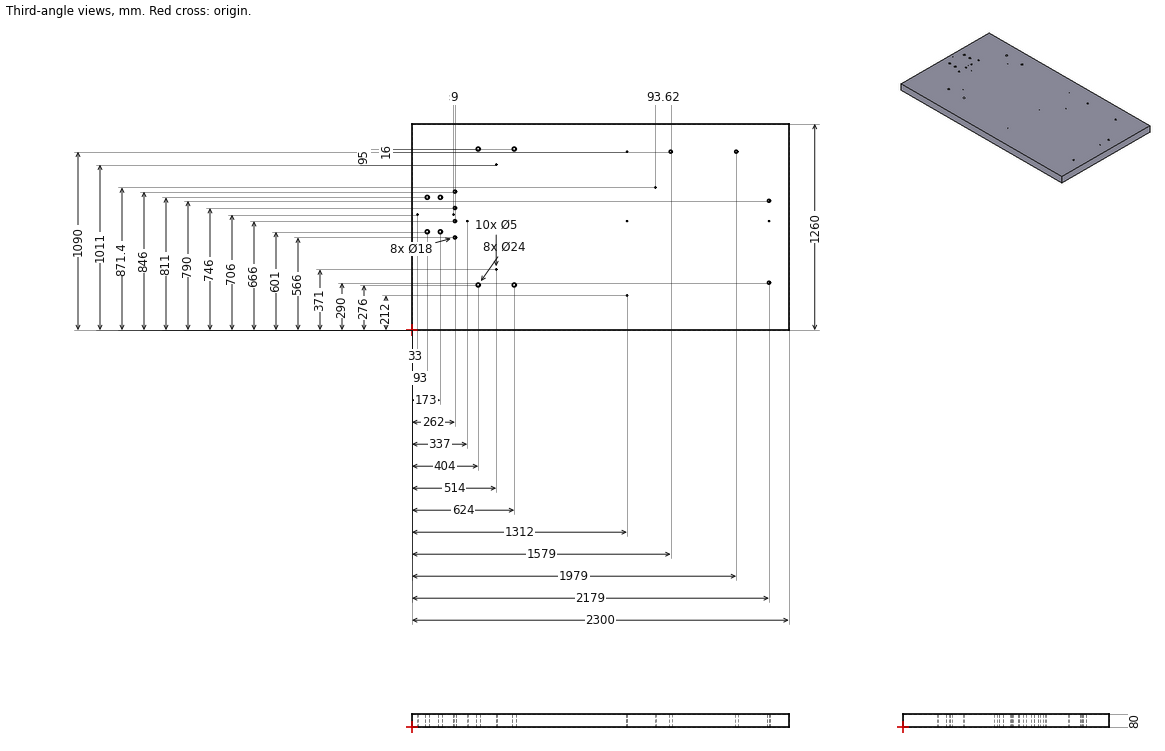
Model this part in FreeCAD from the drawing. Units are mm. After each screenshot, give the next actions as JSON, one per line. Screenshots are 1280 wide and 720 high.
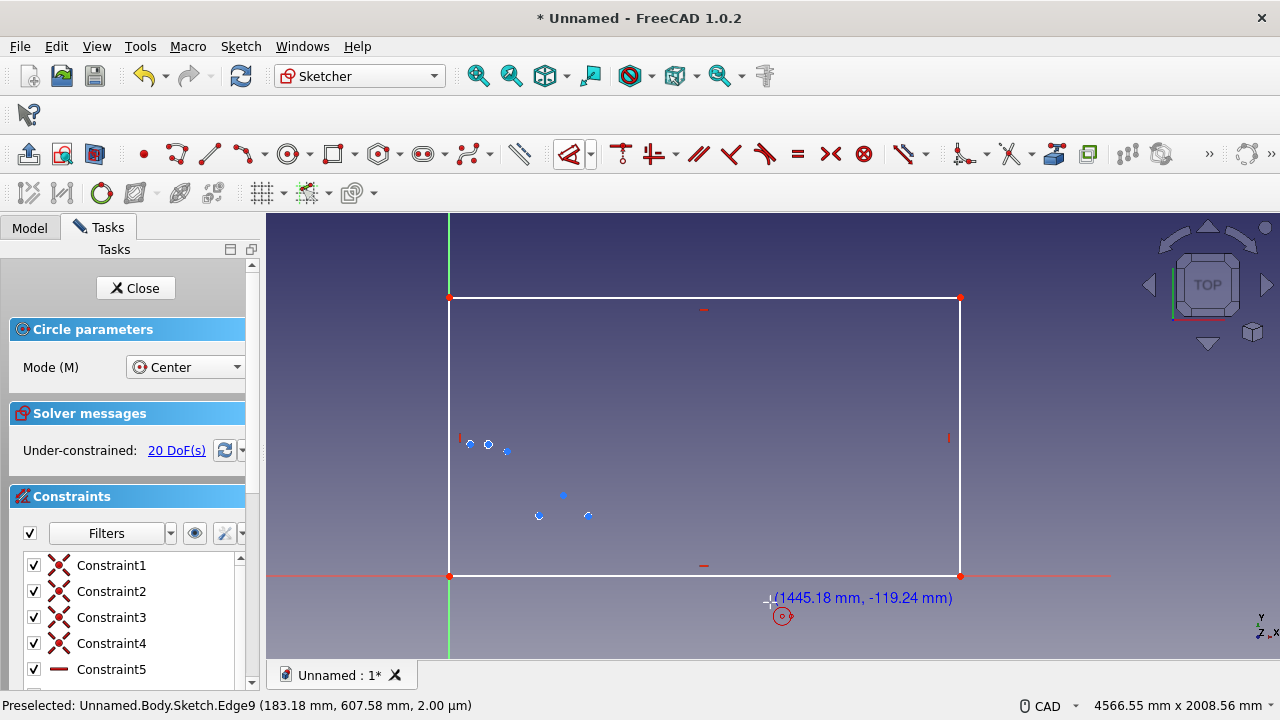
{"action": "left_click", "coordinate": [741, 529]}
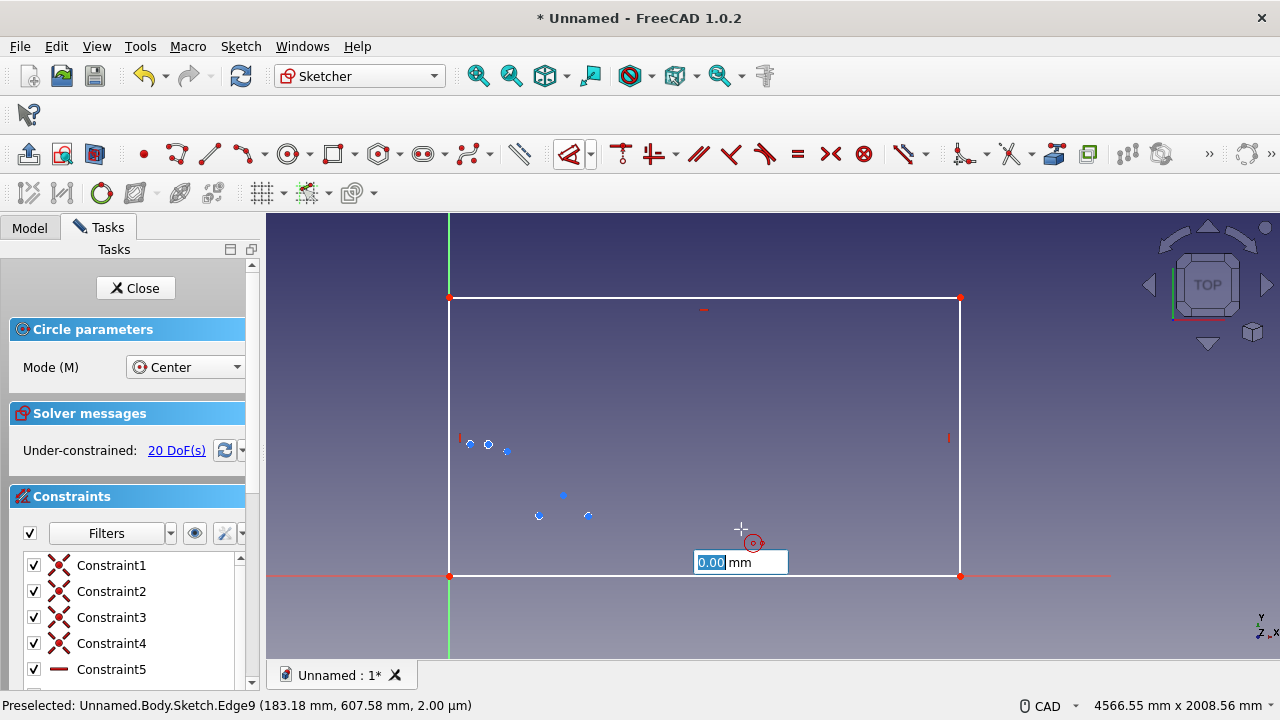
{"action": "scroll", "coordinate": [741, 529], "scroll_direction": "up", "scroll_amount": 17}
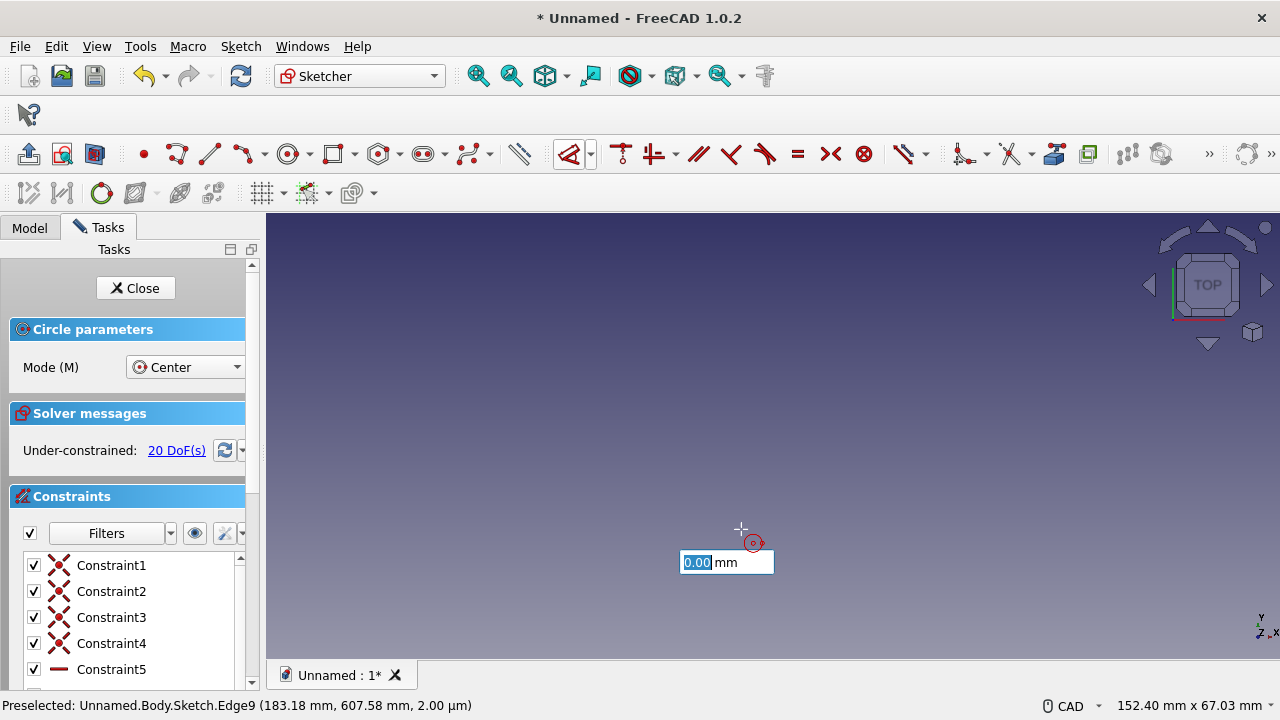
{"action": "left_click", "coordinate": [730, 508]}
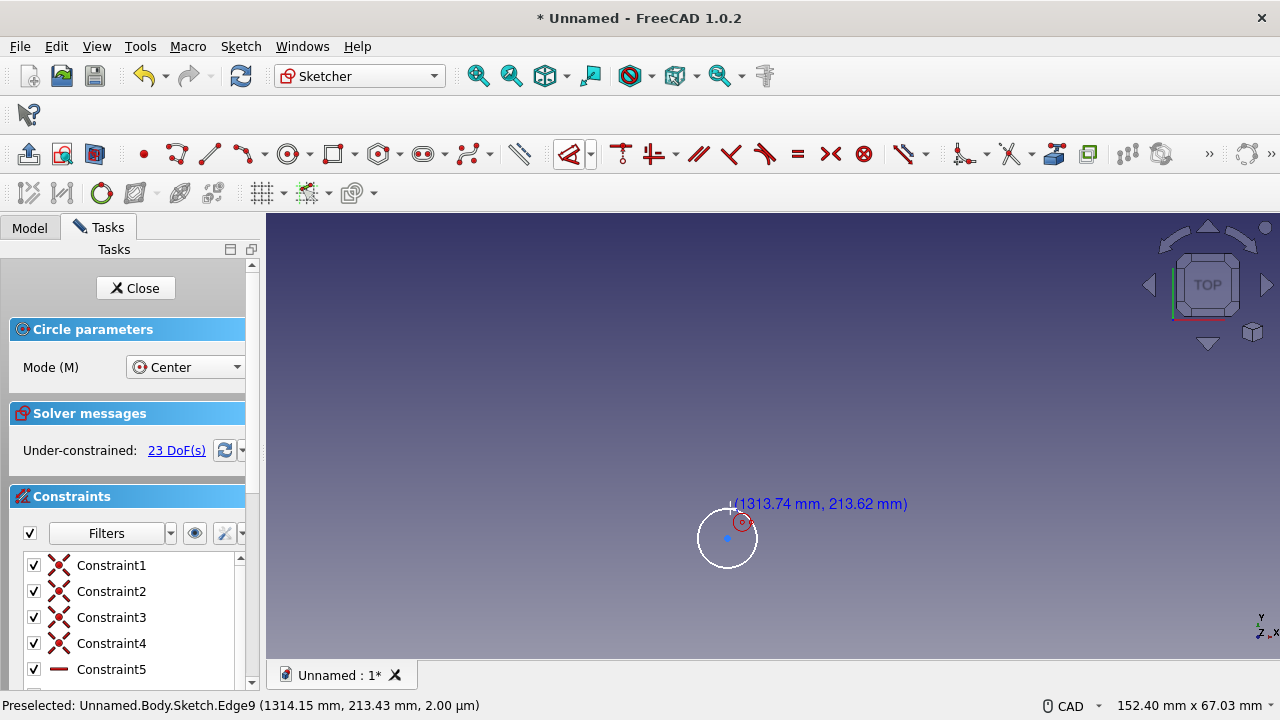
{"action": "scroll", "coordinate": [741, 529], "scroll_direction": "down", "scroll_amount": 17}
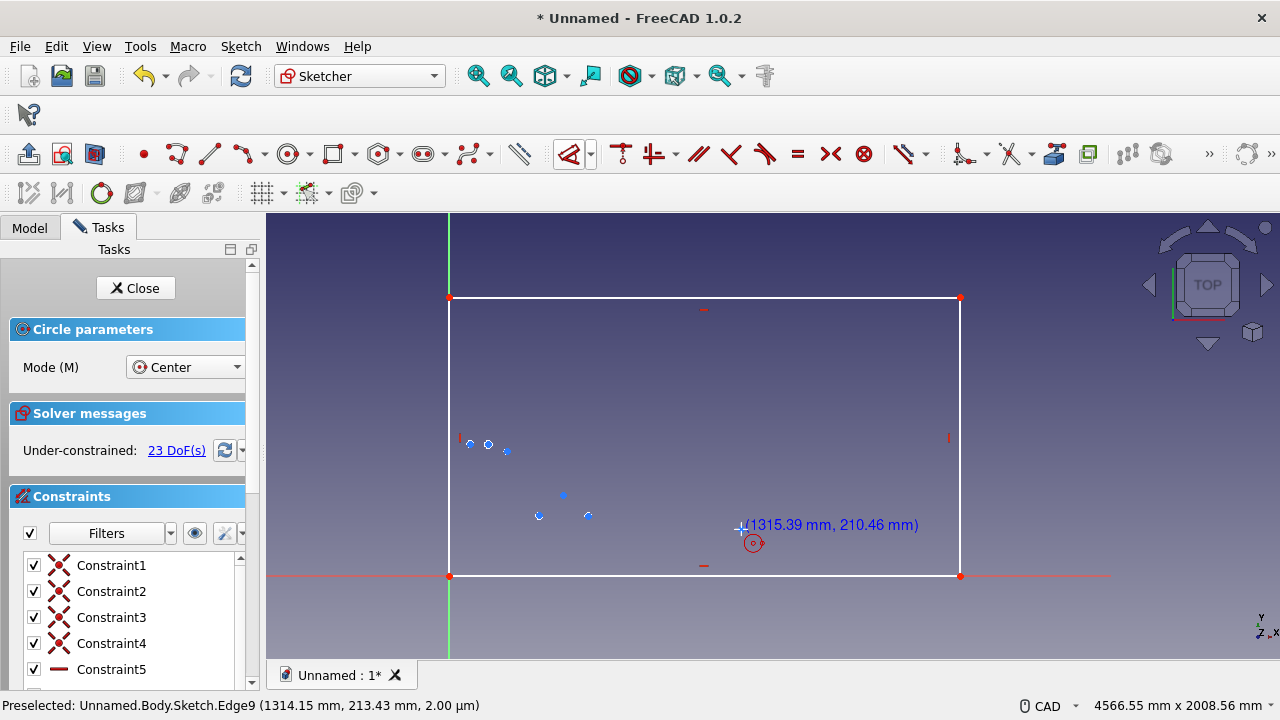
{"action": "scroll", "coordinate": [933, 512], "scroll_direction": "up", "scroll_amount": 13}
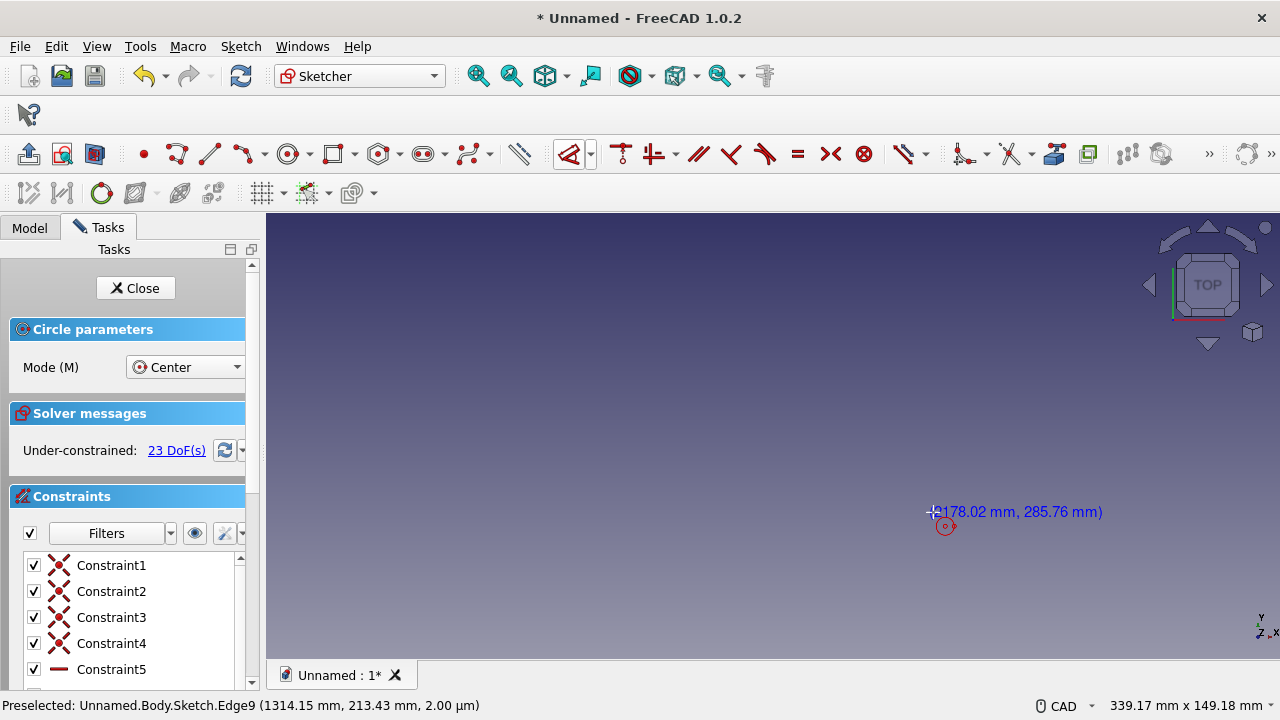
{"action": "scroll", "coordinate": [933, 512], "scroll_direction": "down", "scroll_amount": 13}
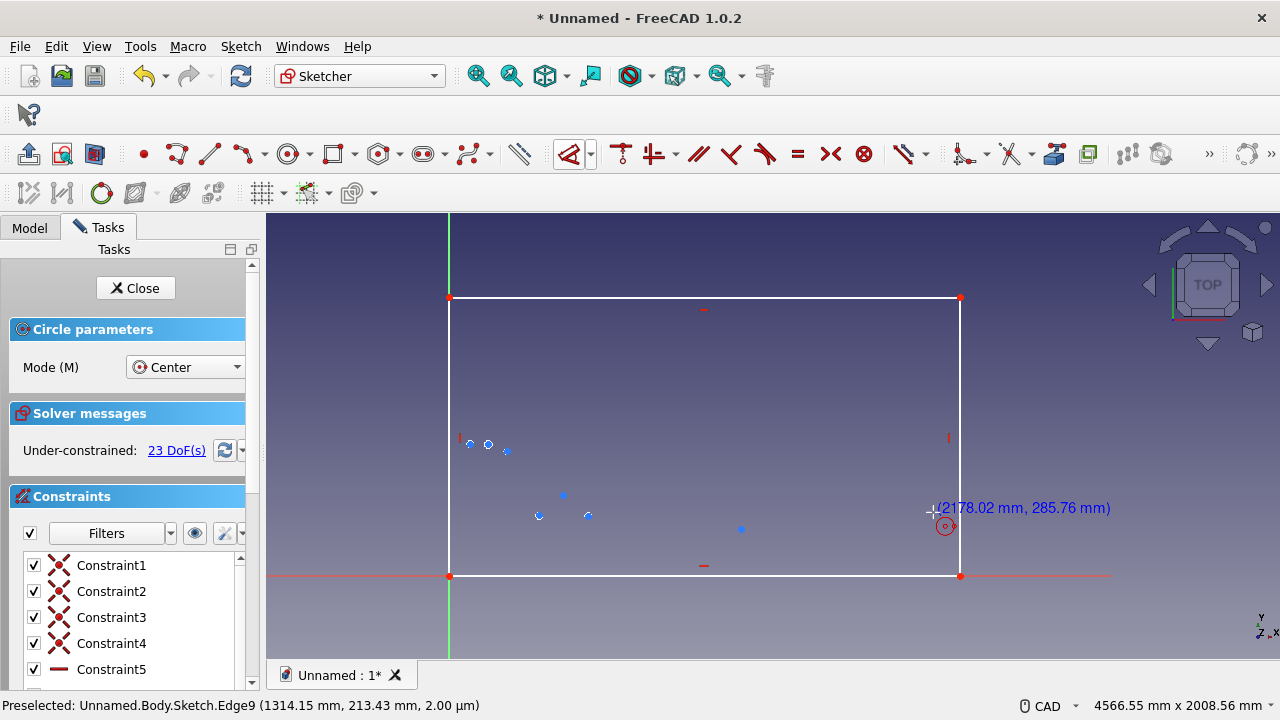
{"action": "left_click", "coordinate": [933, 512]}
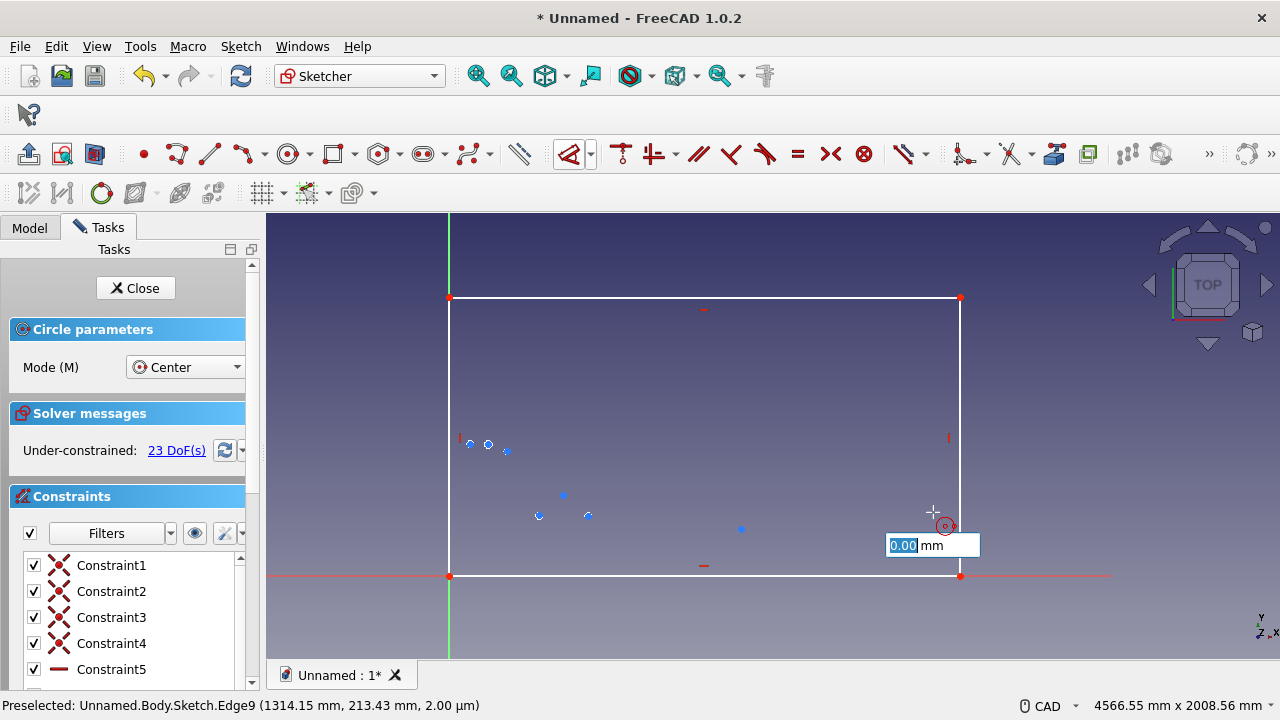
{"action": "scroll", "coordinate": [935, 511], "scroll_direction": "up", "scroll_amount": 11}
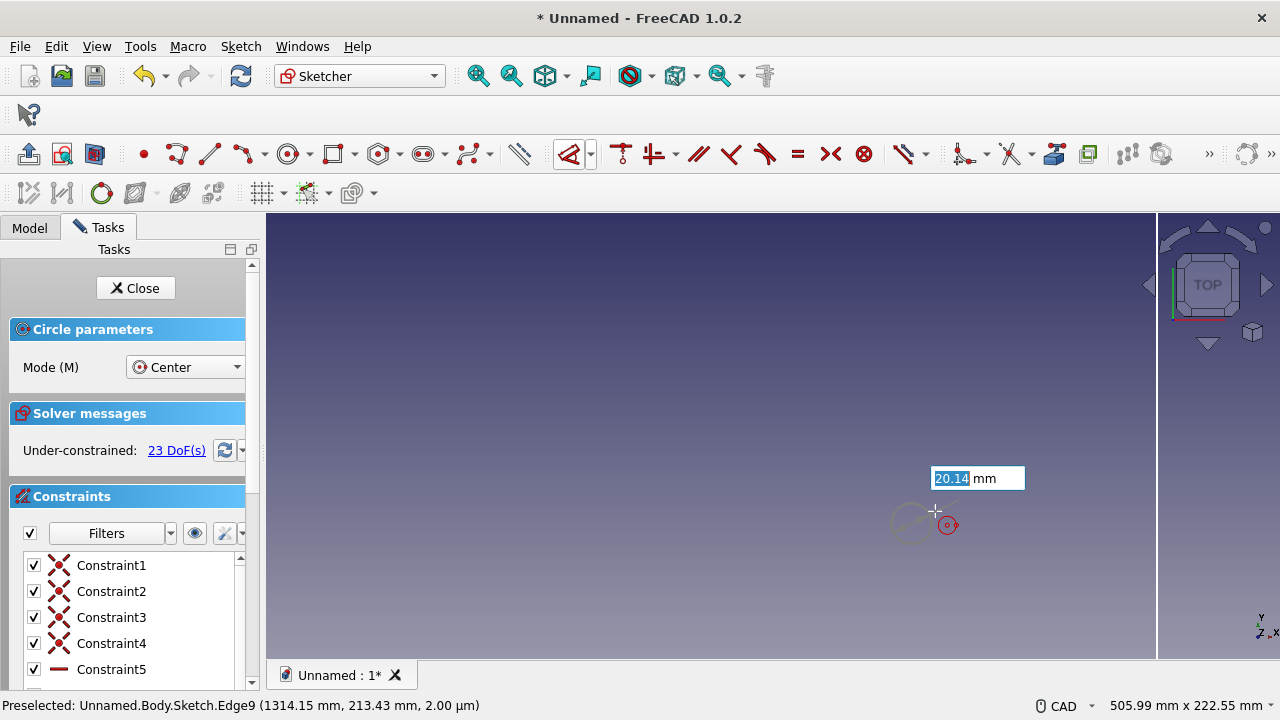
{"action": "left_click", "coordinate": [926, 502]}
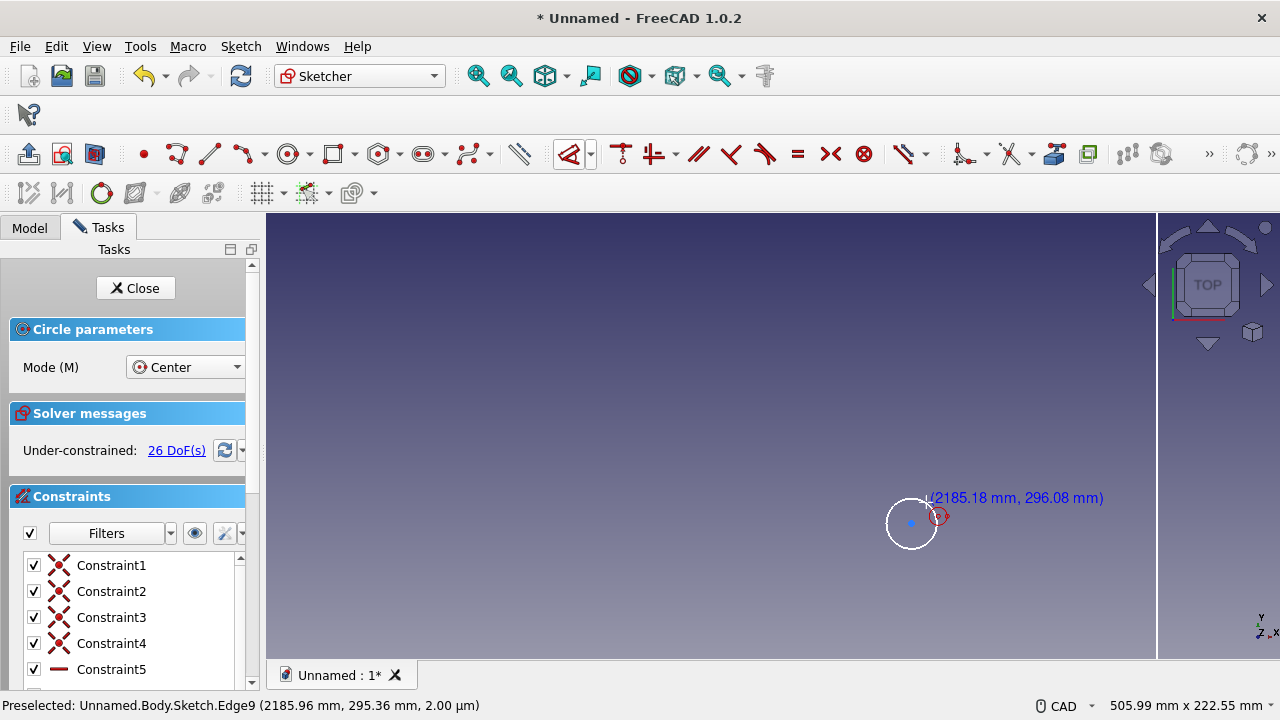
{"action": "scroll", "coordinate": [935, 511], "scroll_direction": "down", "scroll_amount": 11}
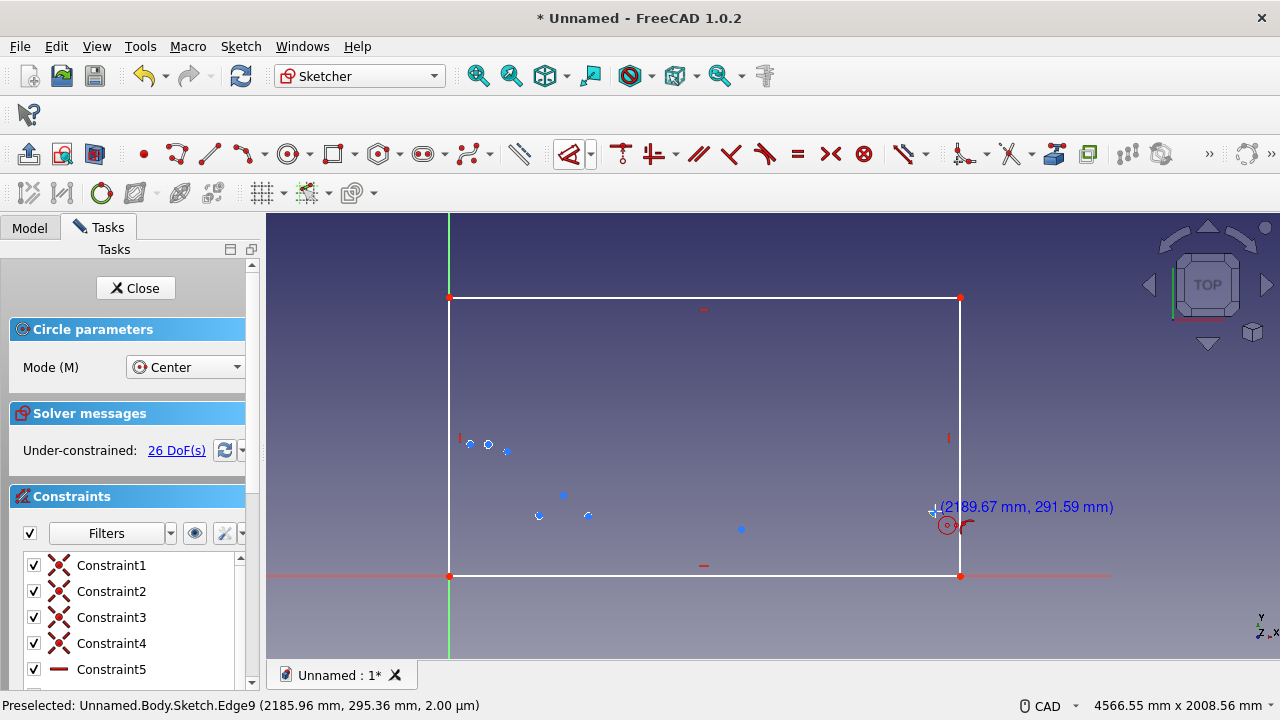
{"action": "scroll", "coordinate": [457, 420], "scroll_direction": "up", "scroll_amount": 19}